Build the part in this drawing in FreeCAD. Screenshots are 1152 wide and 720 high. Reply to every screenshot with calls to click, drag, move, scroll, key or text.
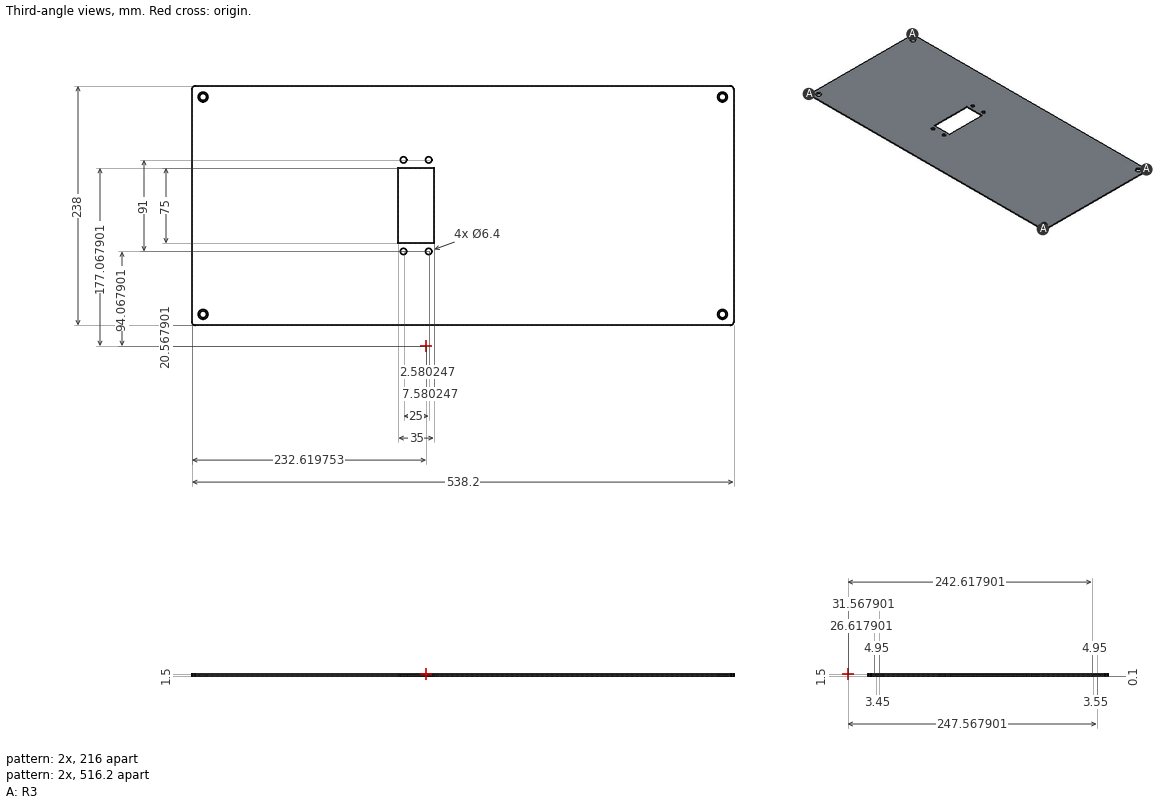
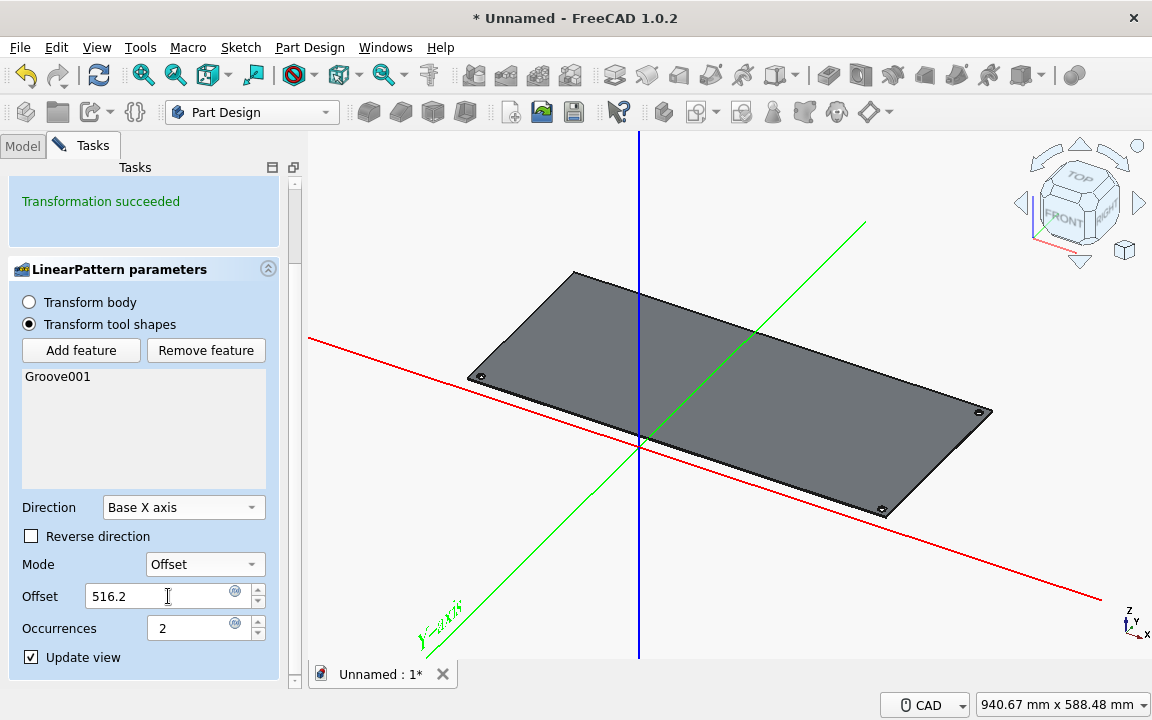
triple_click(198, 628)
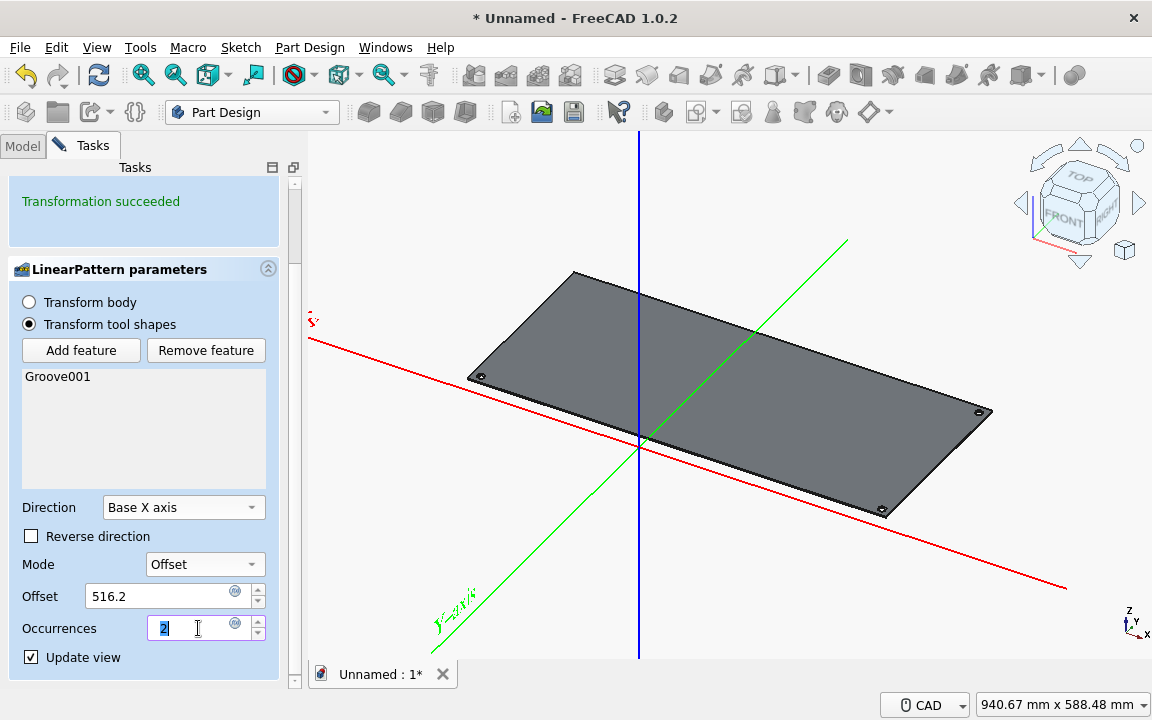
text(2)
key(Tab)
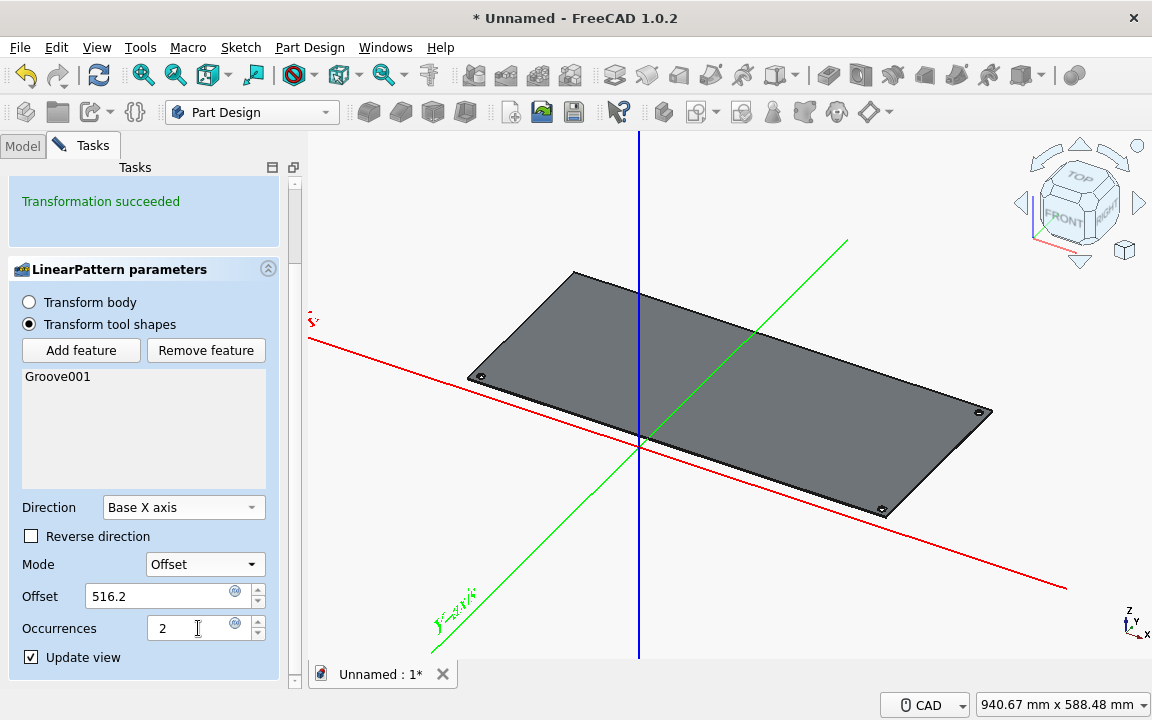
click(30, 536)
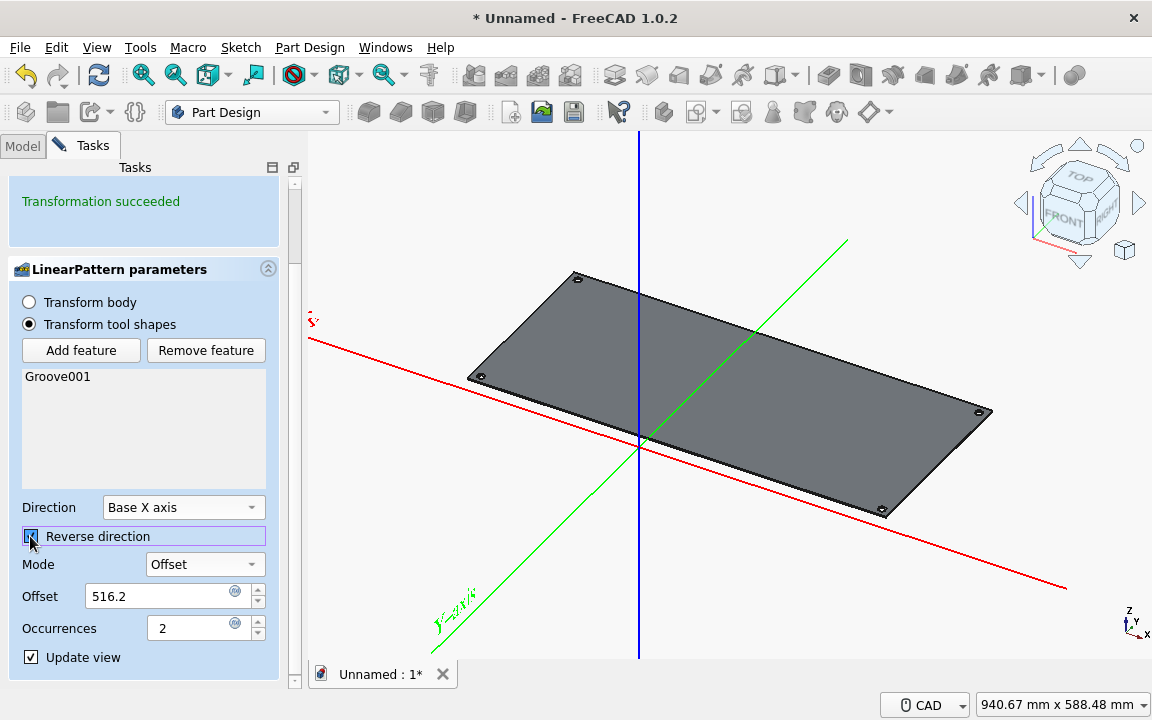
scroll(295, 432, up, 3)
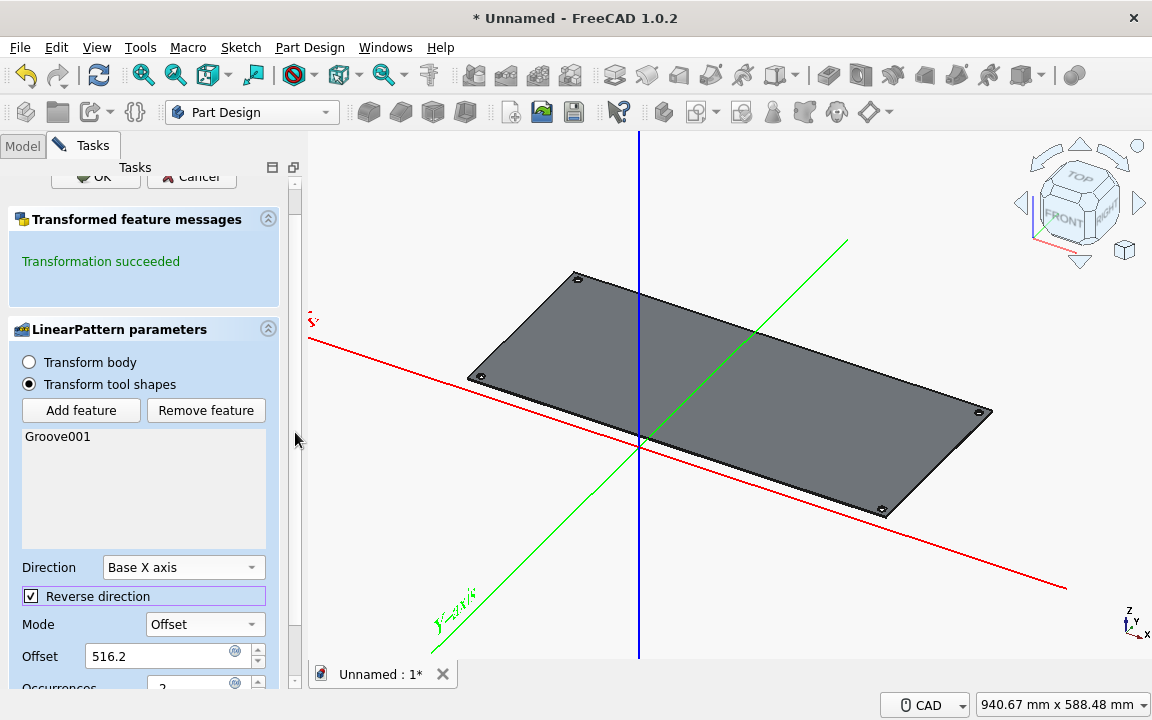
click(96, 206)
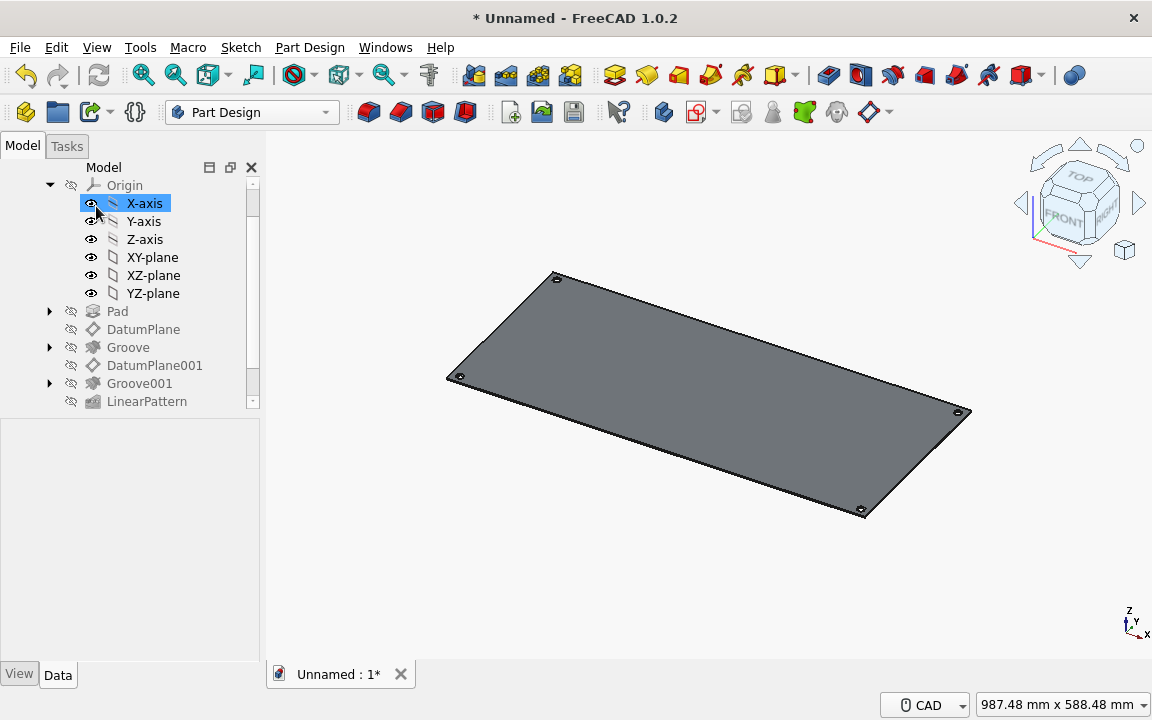
scroll(553, 272, up, 15)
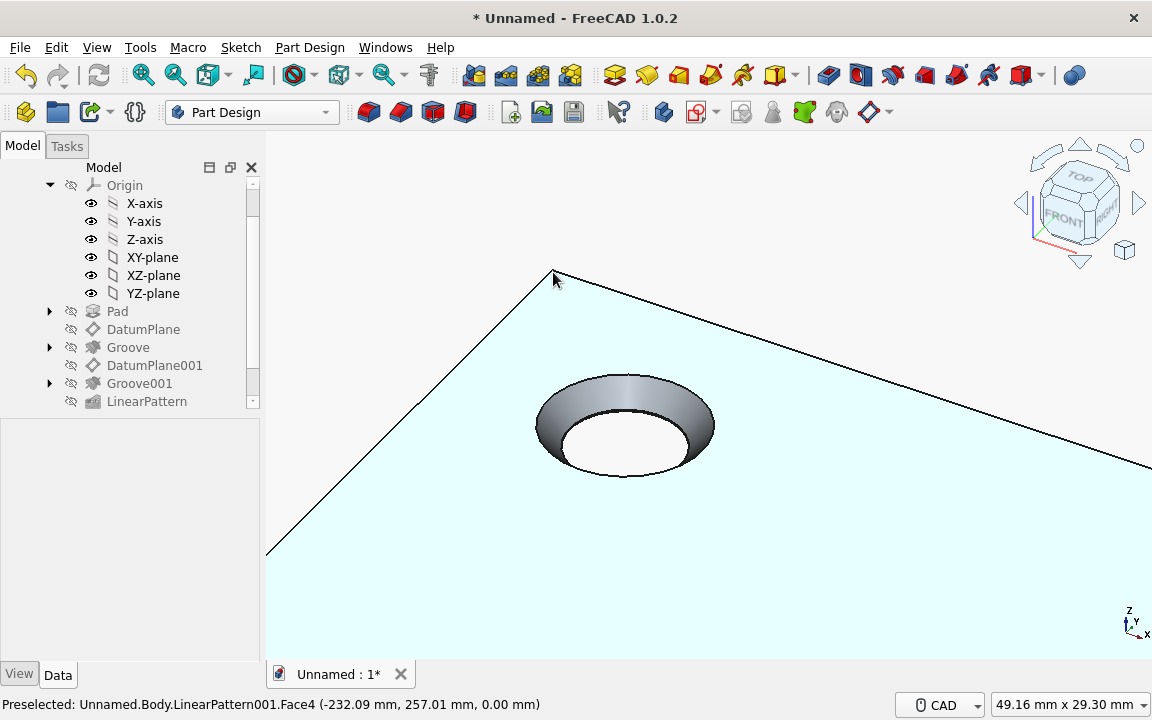
click(144, 76)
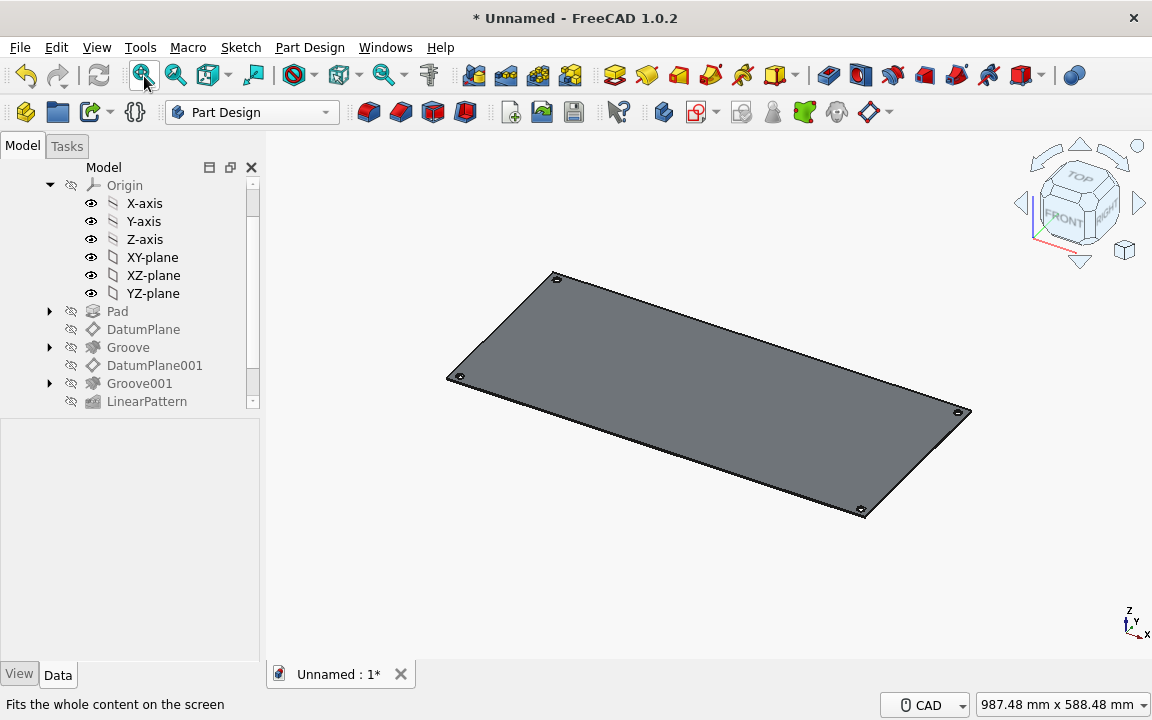
key(0)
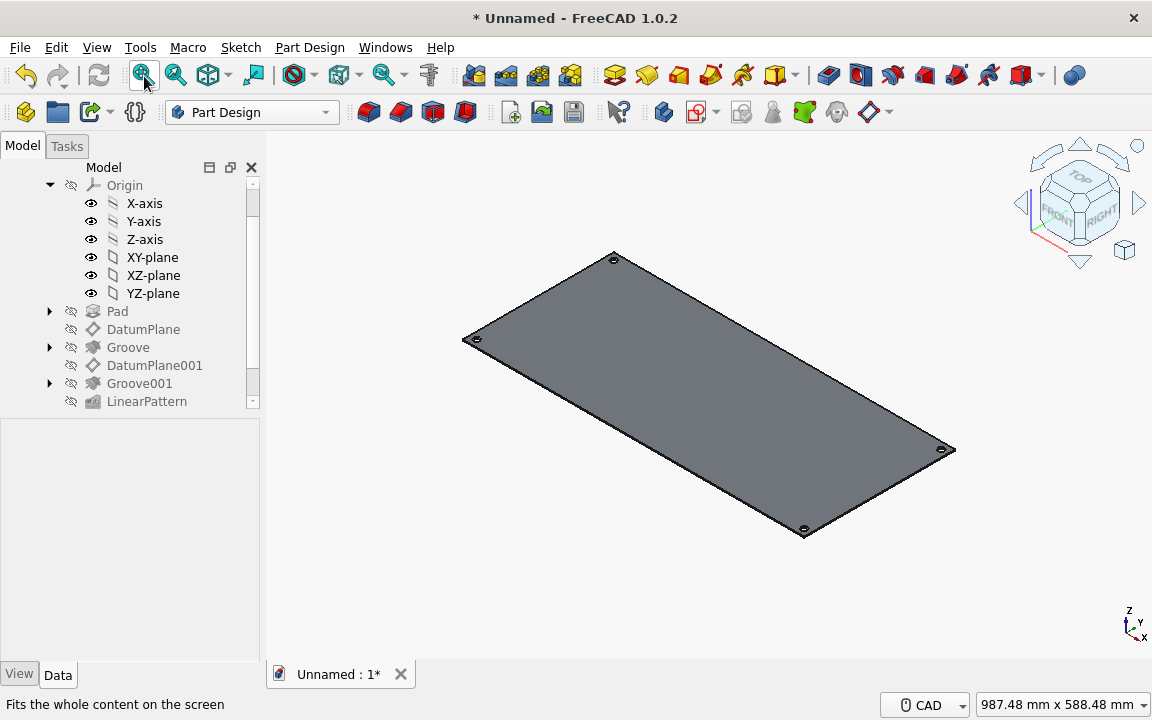
scroll(614, 252, up, 15)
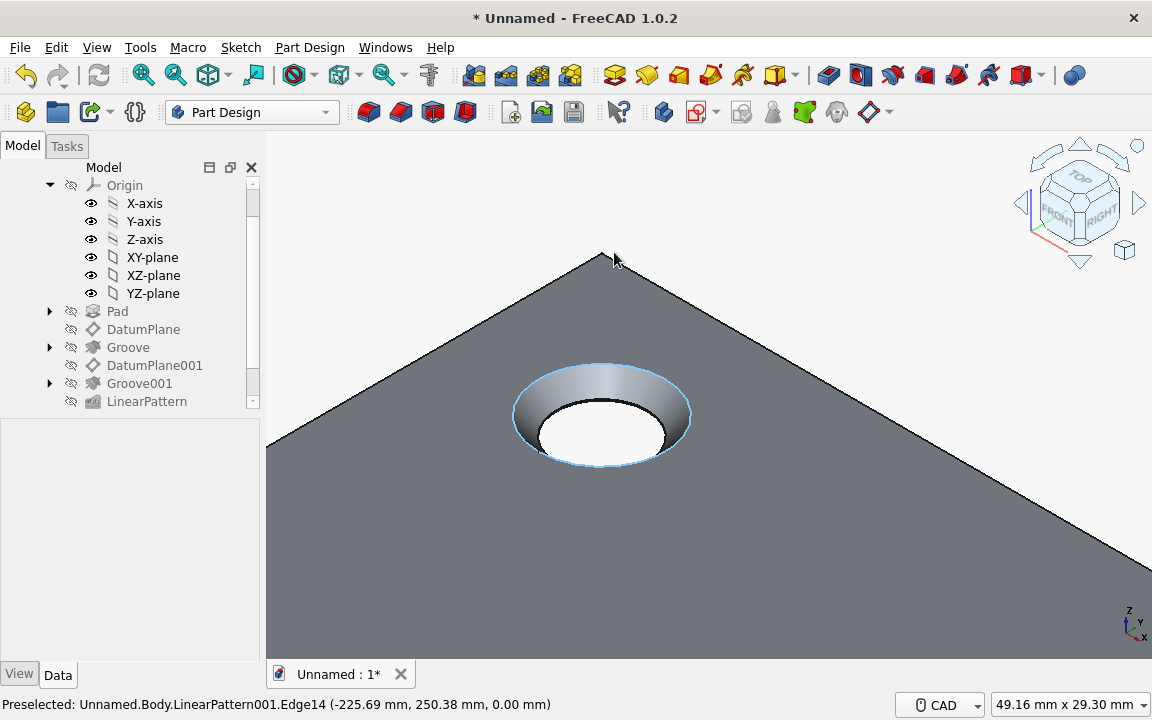
click(144, 76)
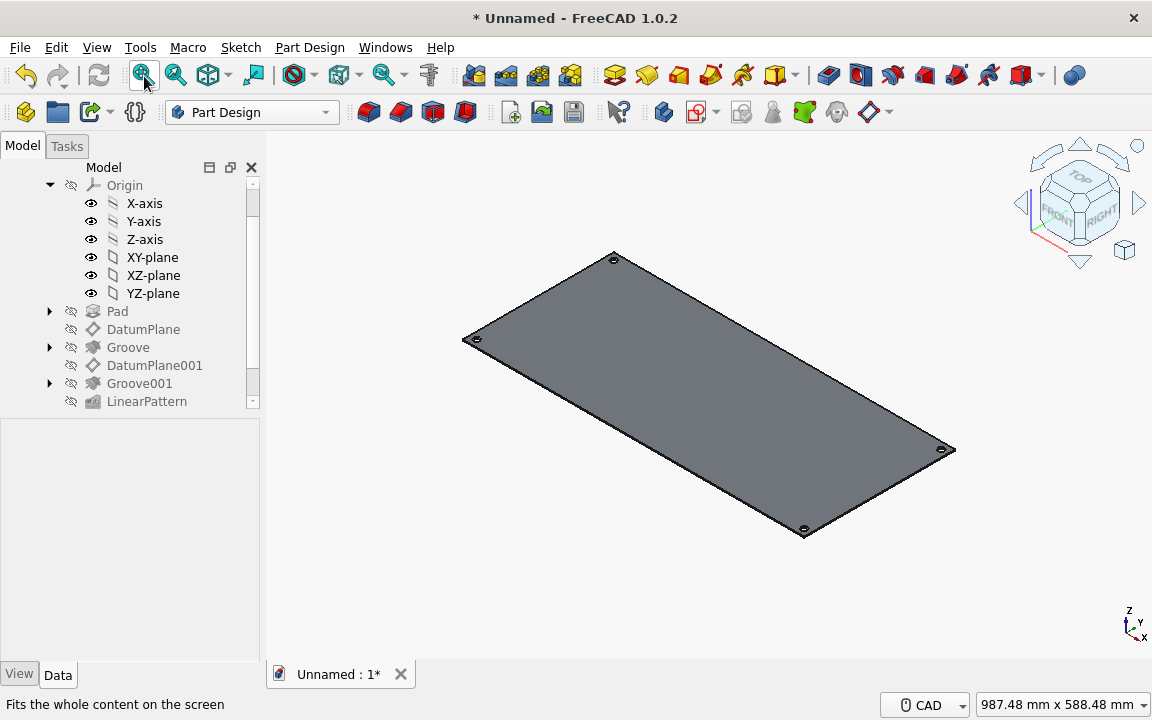
key(2)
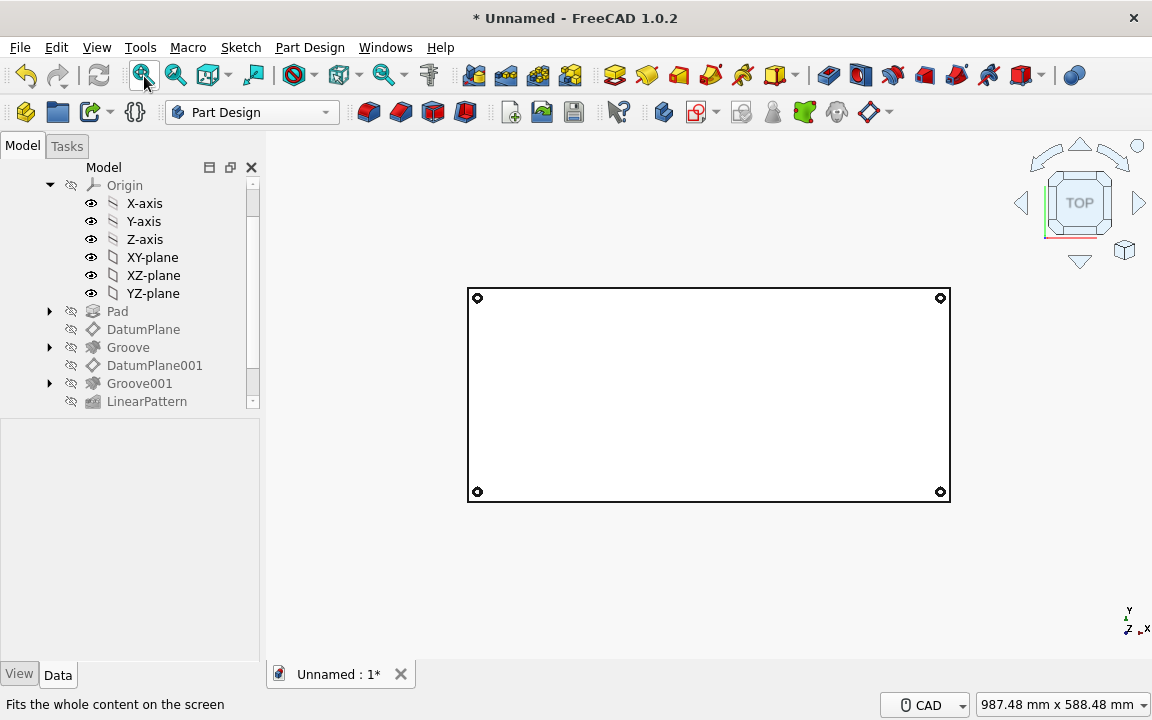
scroll(468, 287, up, 15)